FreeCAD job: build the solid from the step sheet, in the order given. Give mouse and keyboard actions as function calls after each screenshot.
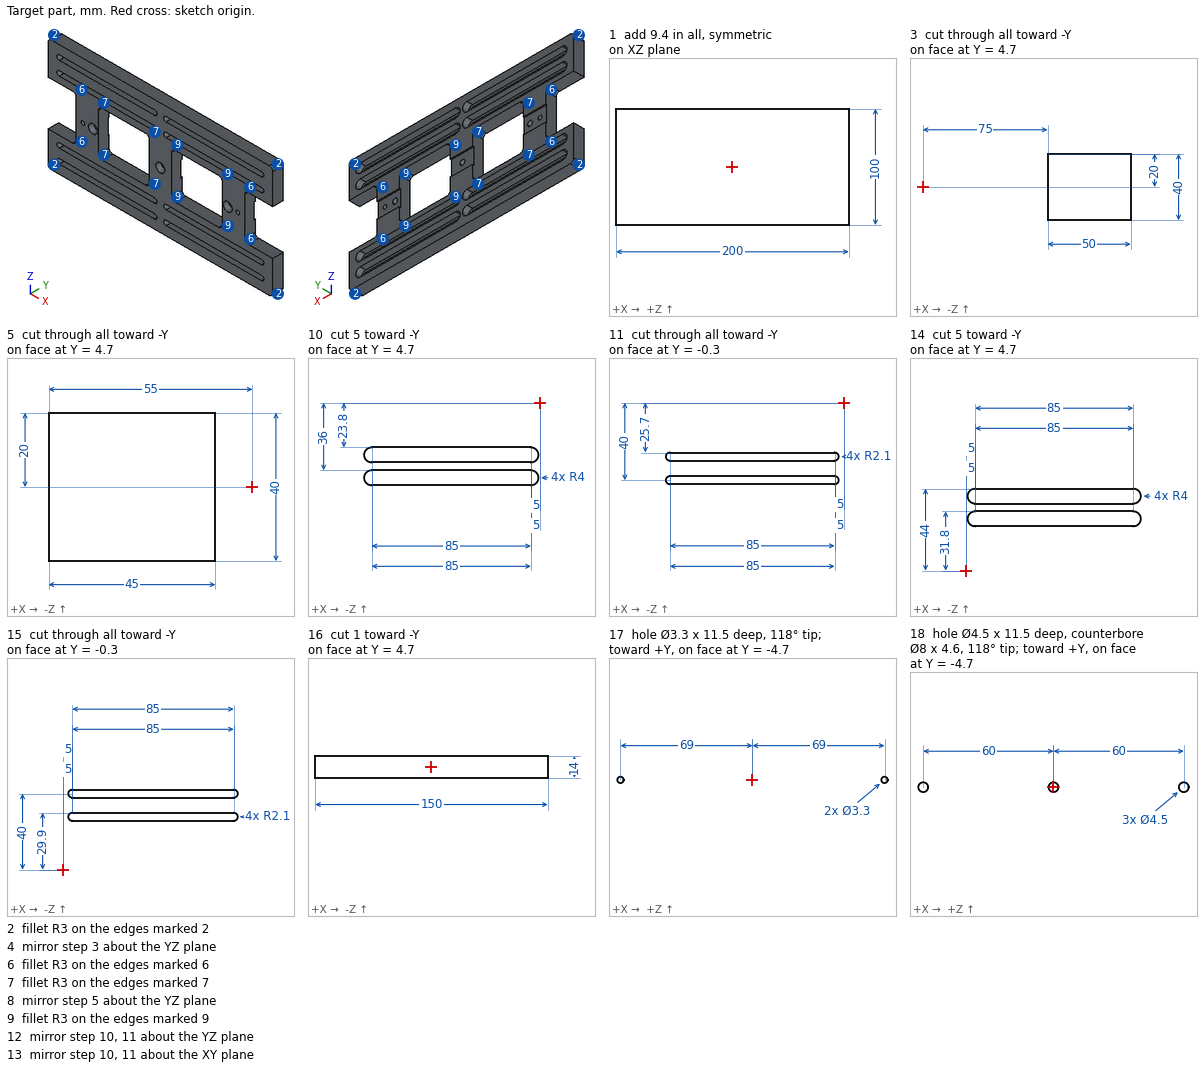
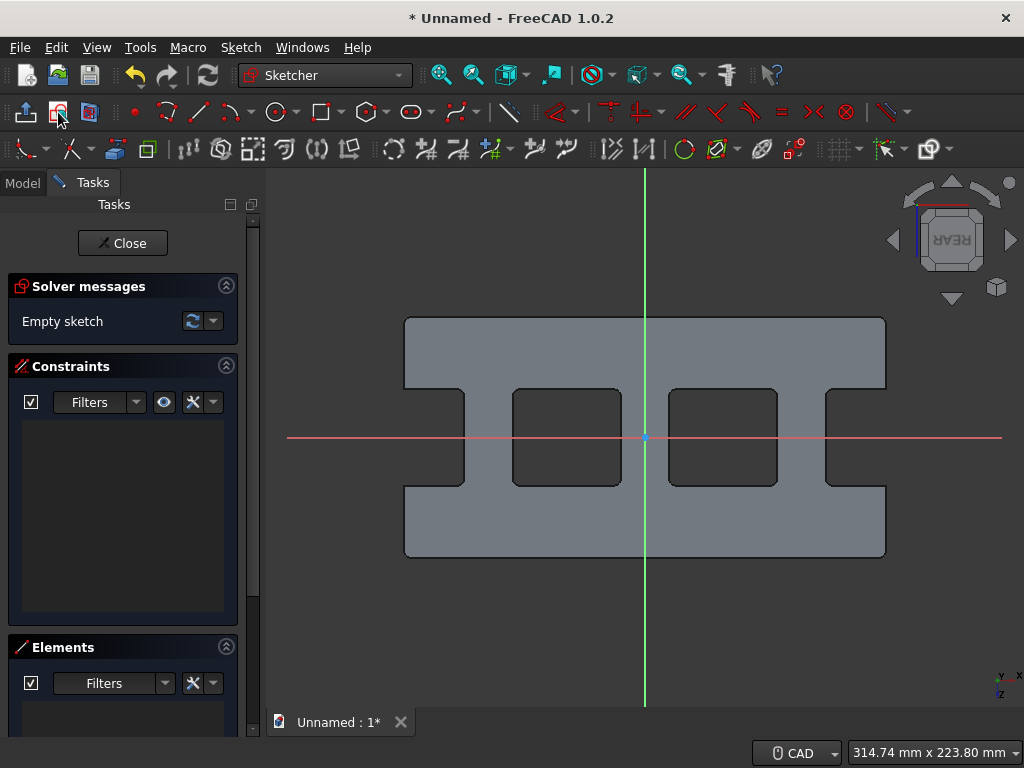
scroll(477, 555, up, 3)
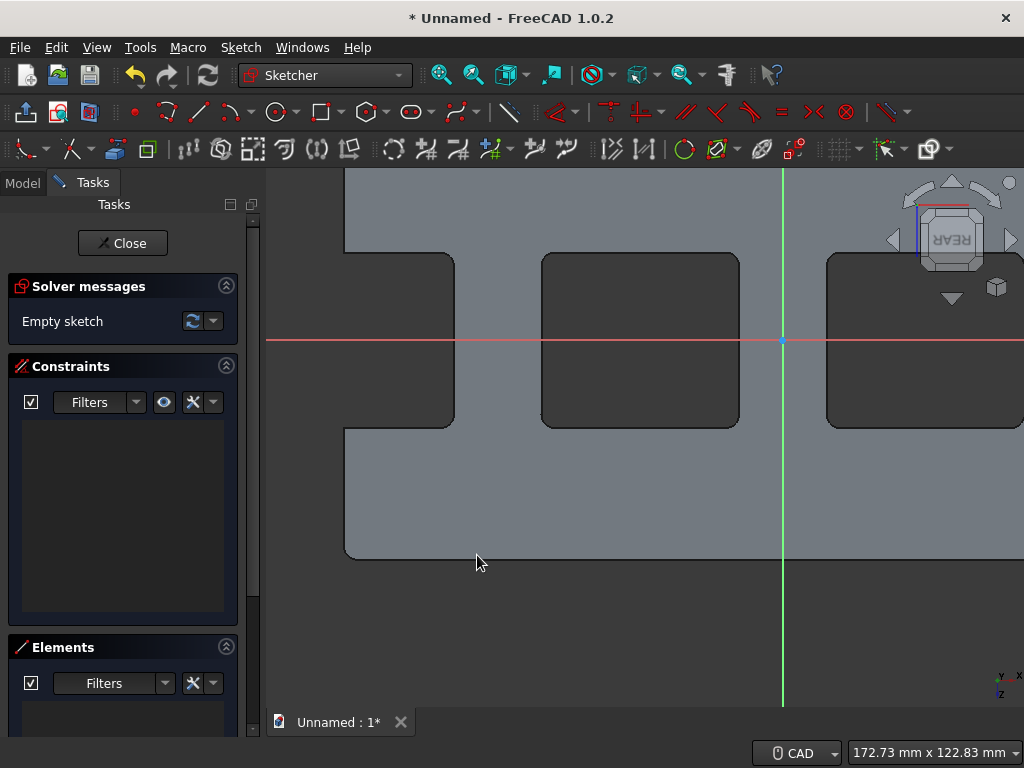
click(412, 112)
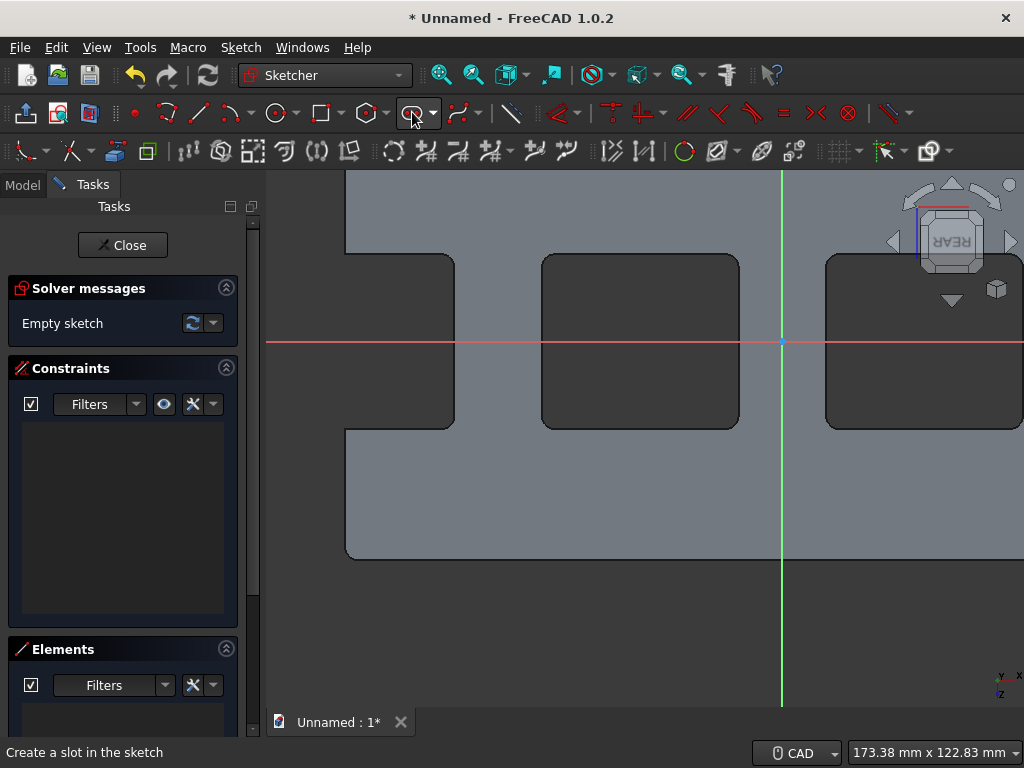
scroll(389, 517, up, 2)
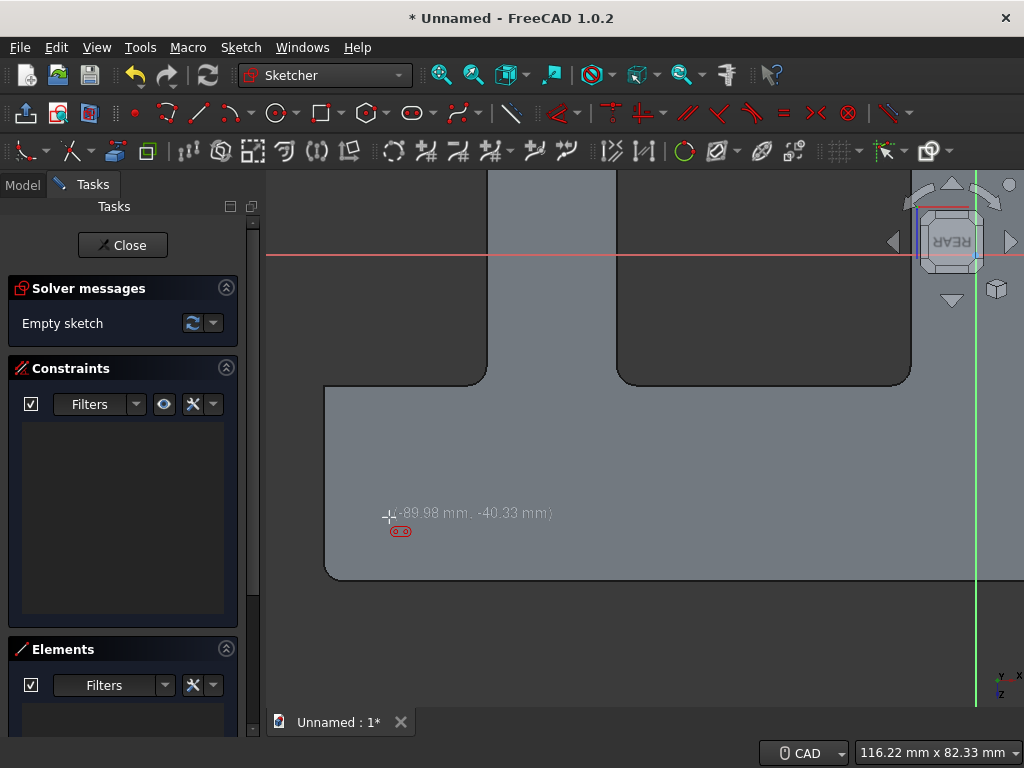
click(389, 516)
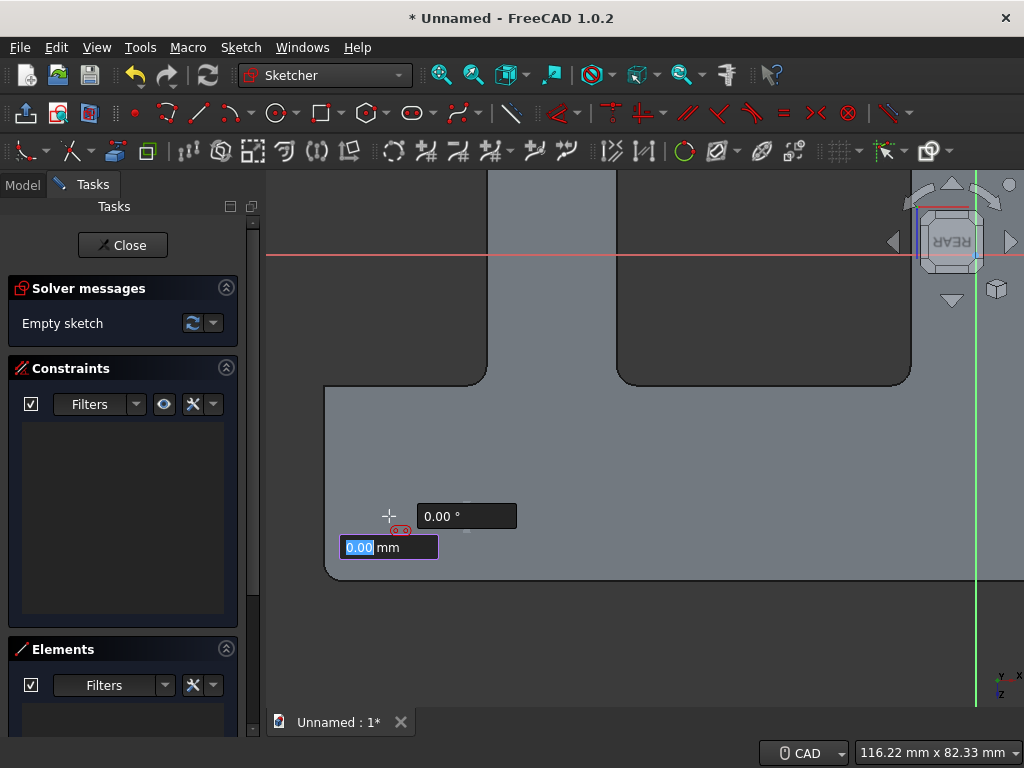
scroll(388, 520, down, 2)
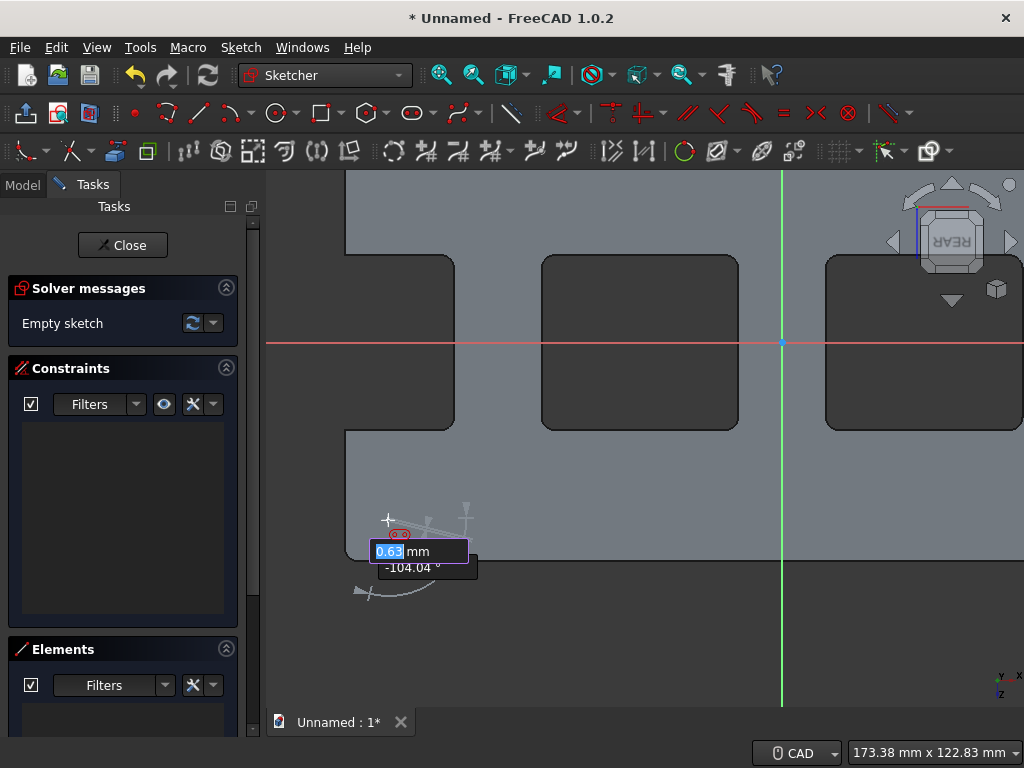
click(760, 518)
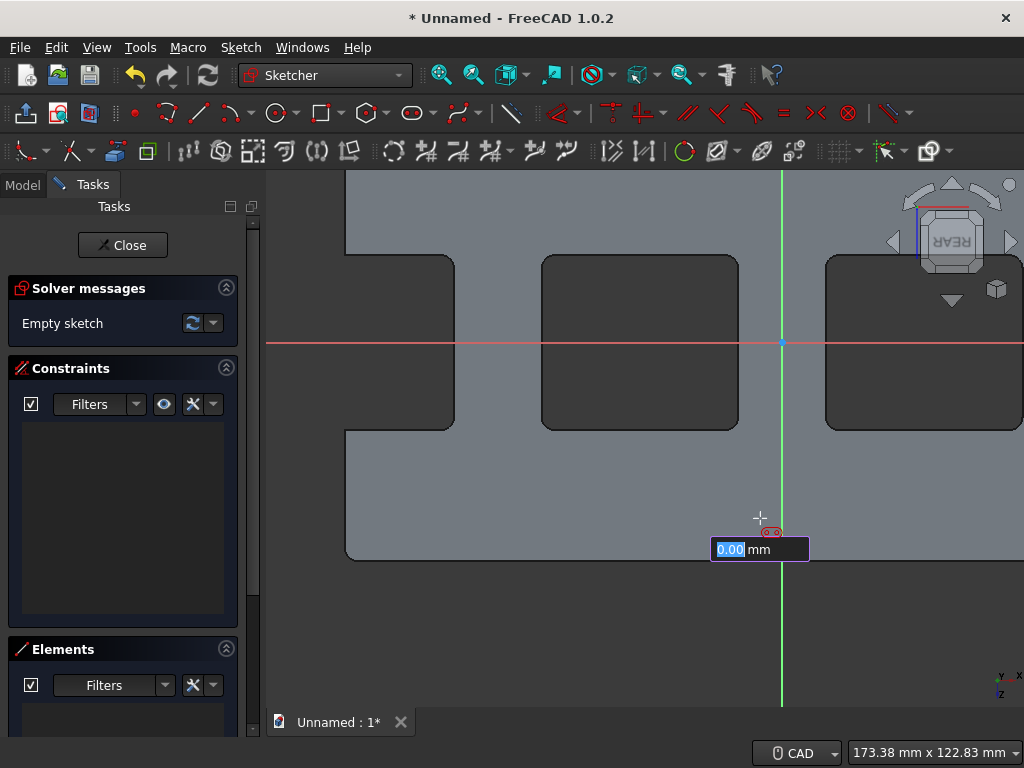
click(574, 500)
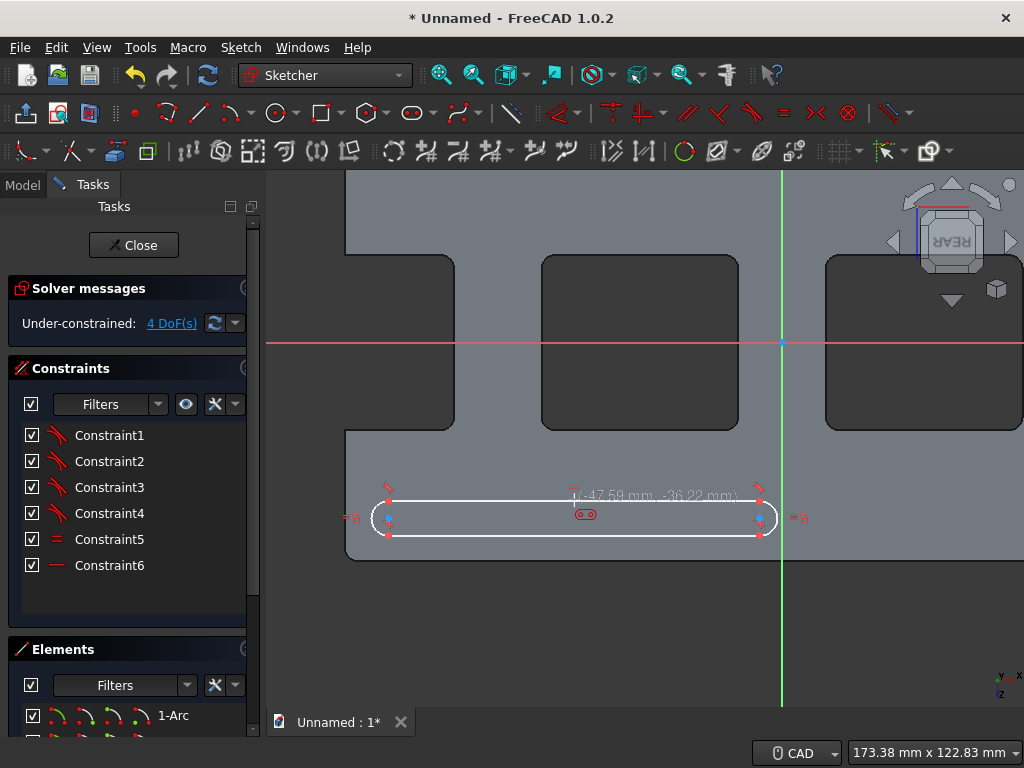
scroll(389, 464, up, 2)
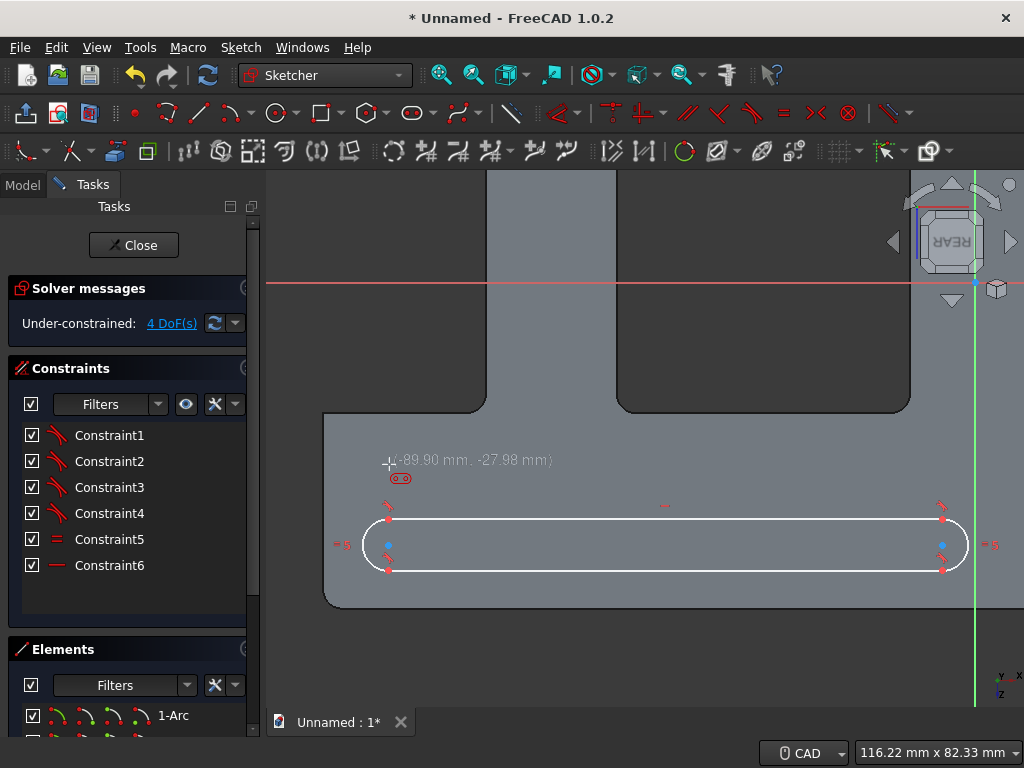
click(388, 464)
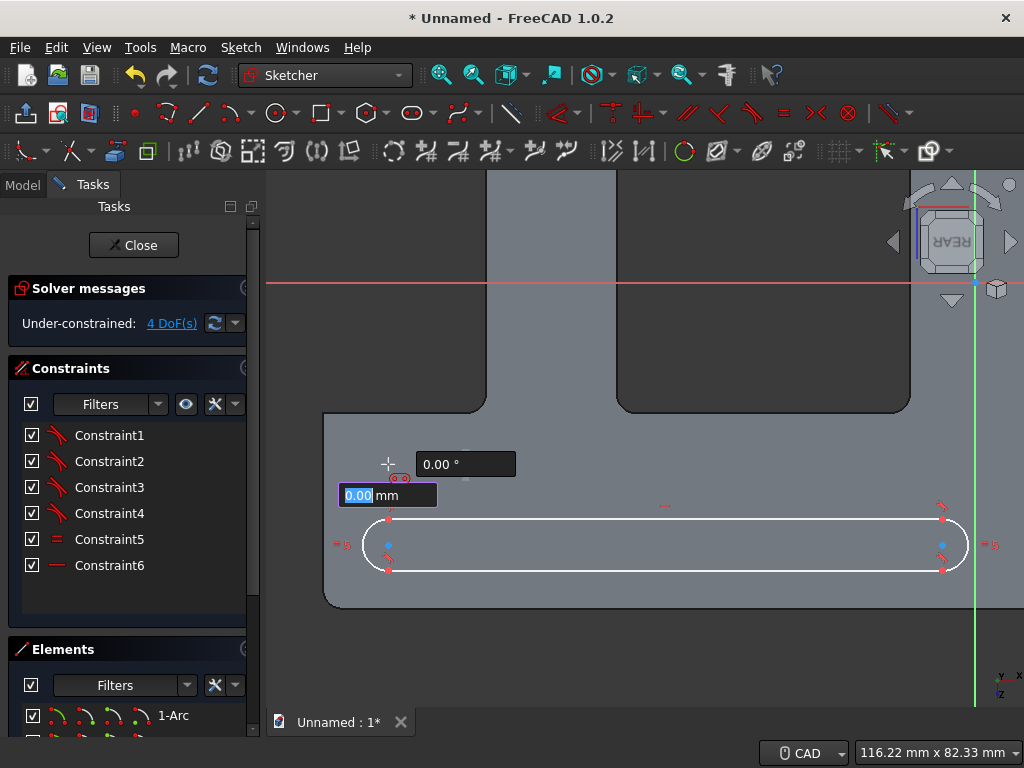
scroll(389, 463, down, 2)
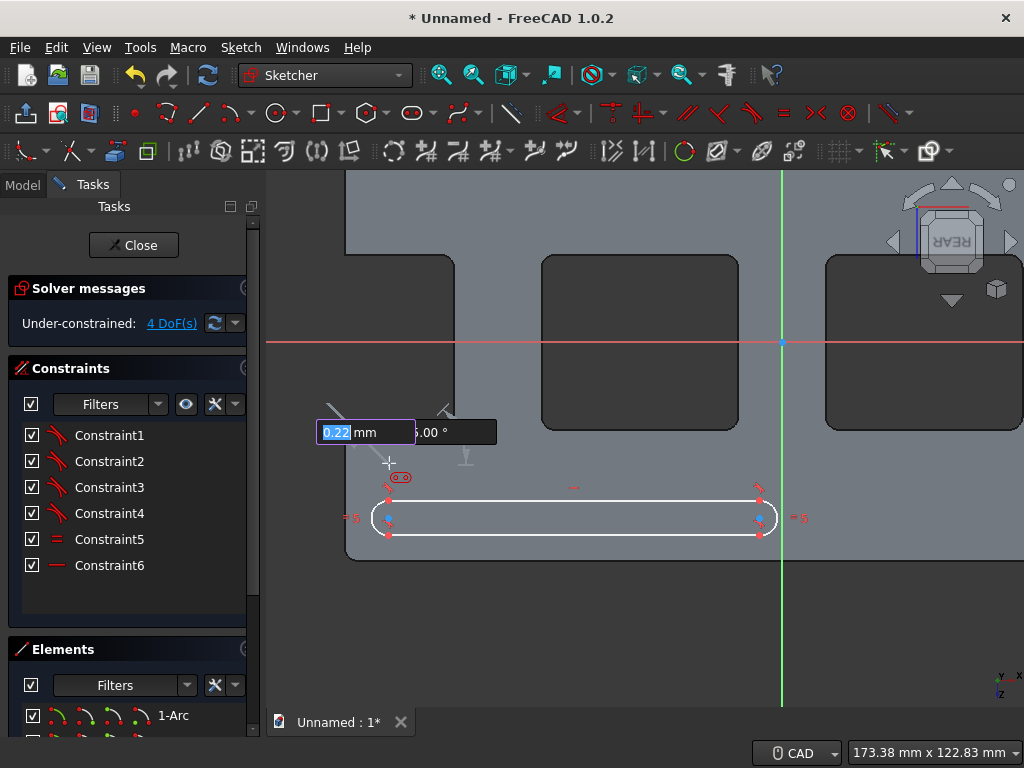
click(760, 464)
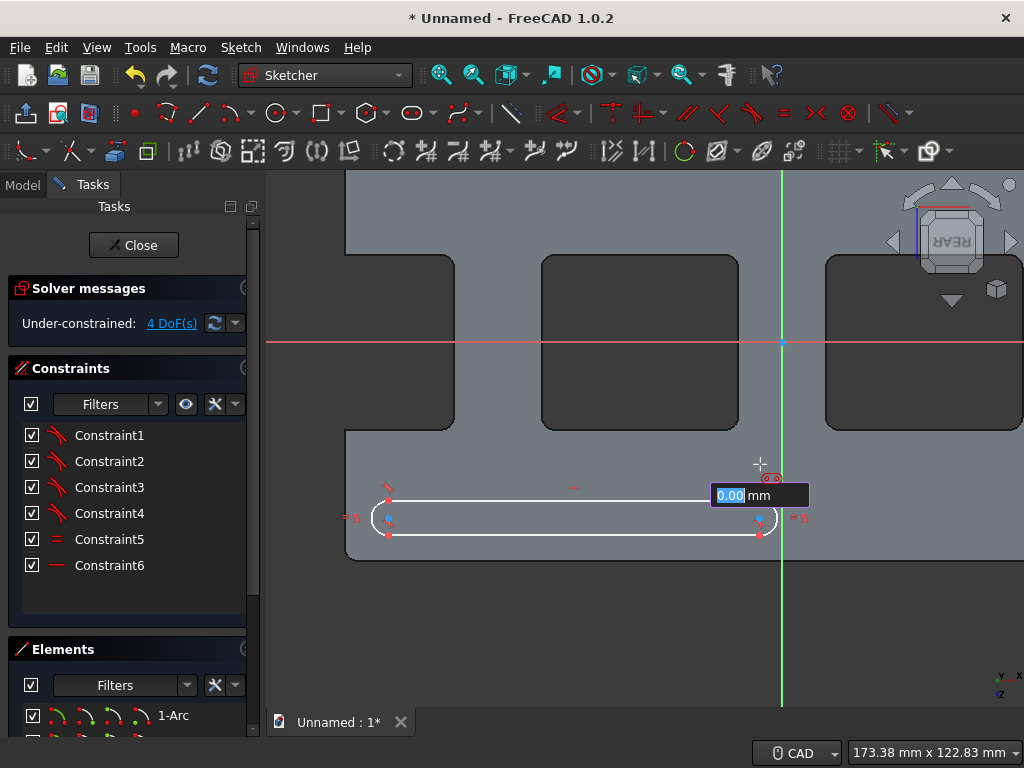
click(574, 481)
key(Escape)